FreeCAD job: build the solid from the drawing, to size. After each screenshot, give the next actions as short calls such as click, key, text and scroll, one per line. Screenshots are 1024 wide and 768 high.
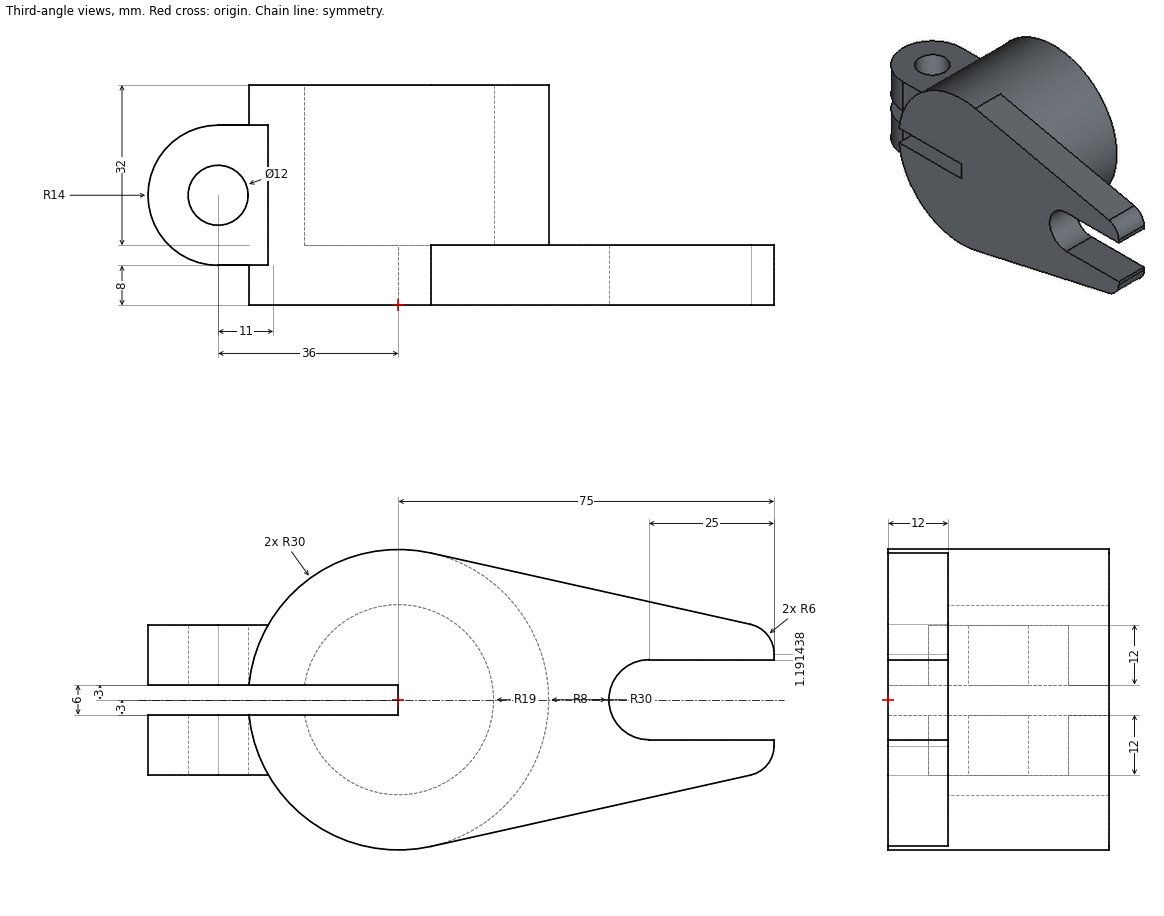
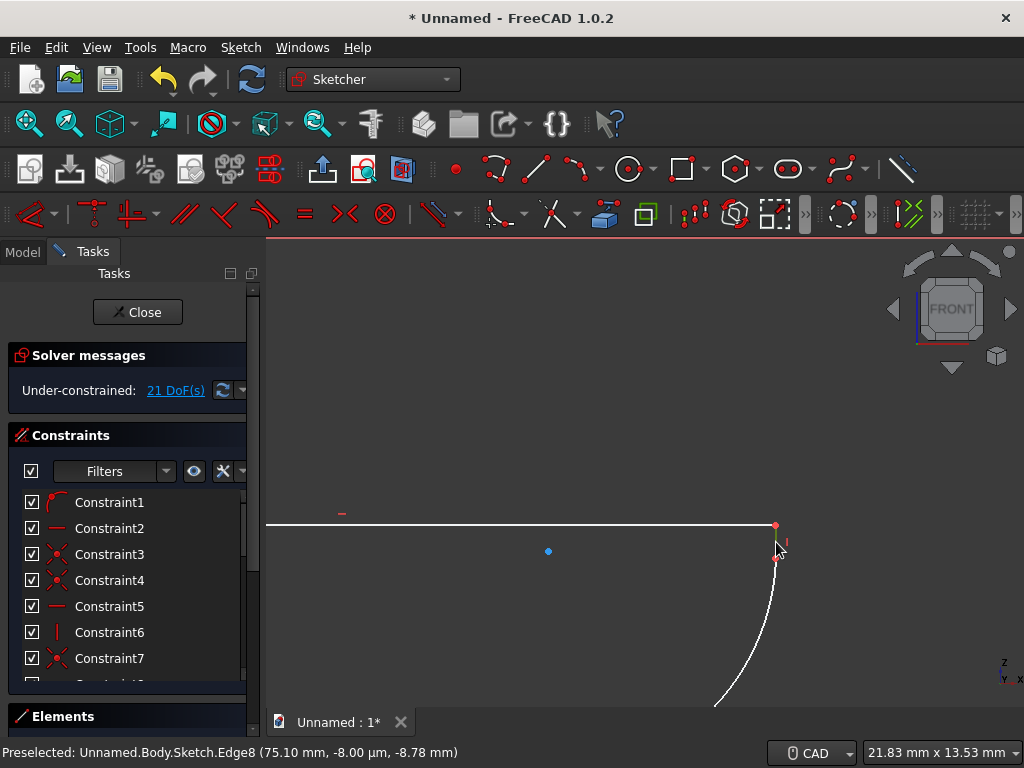
scroll(779, 501, down, 11)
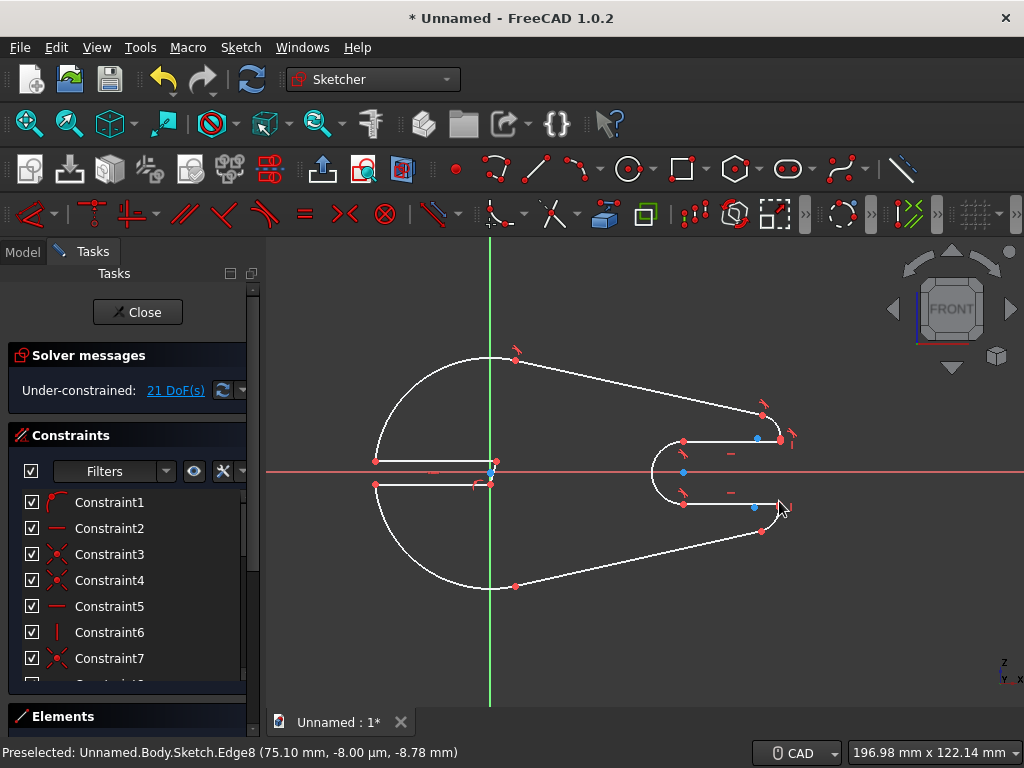
scroll(777, 517, up, 2)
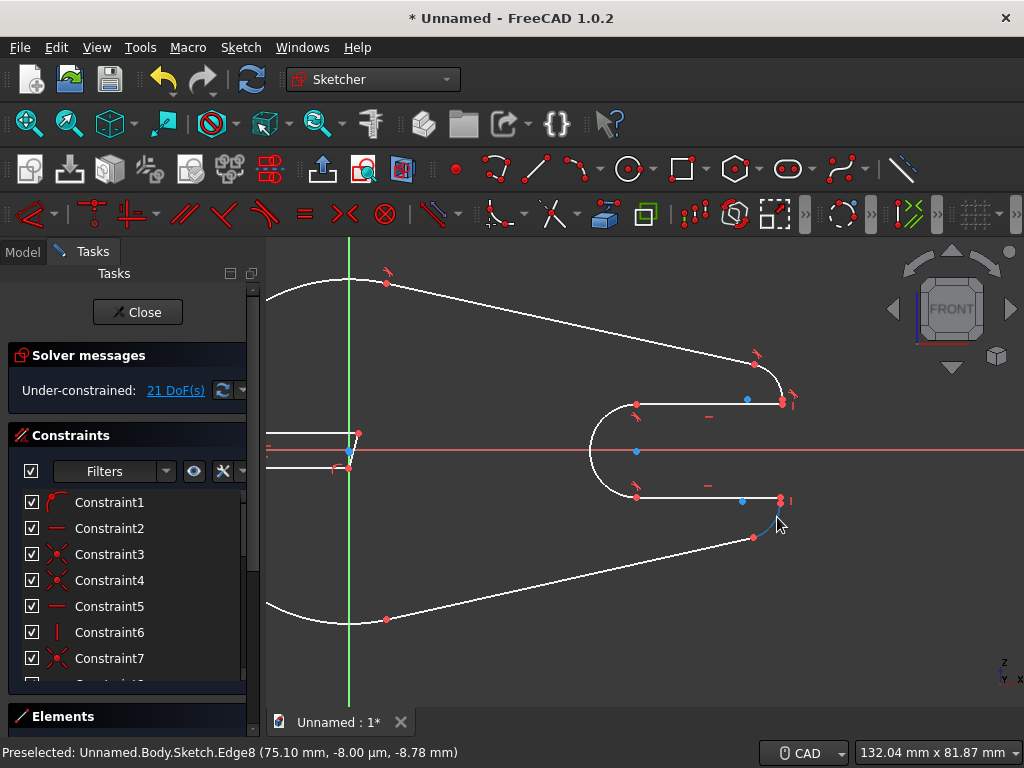
click(777, 517)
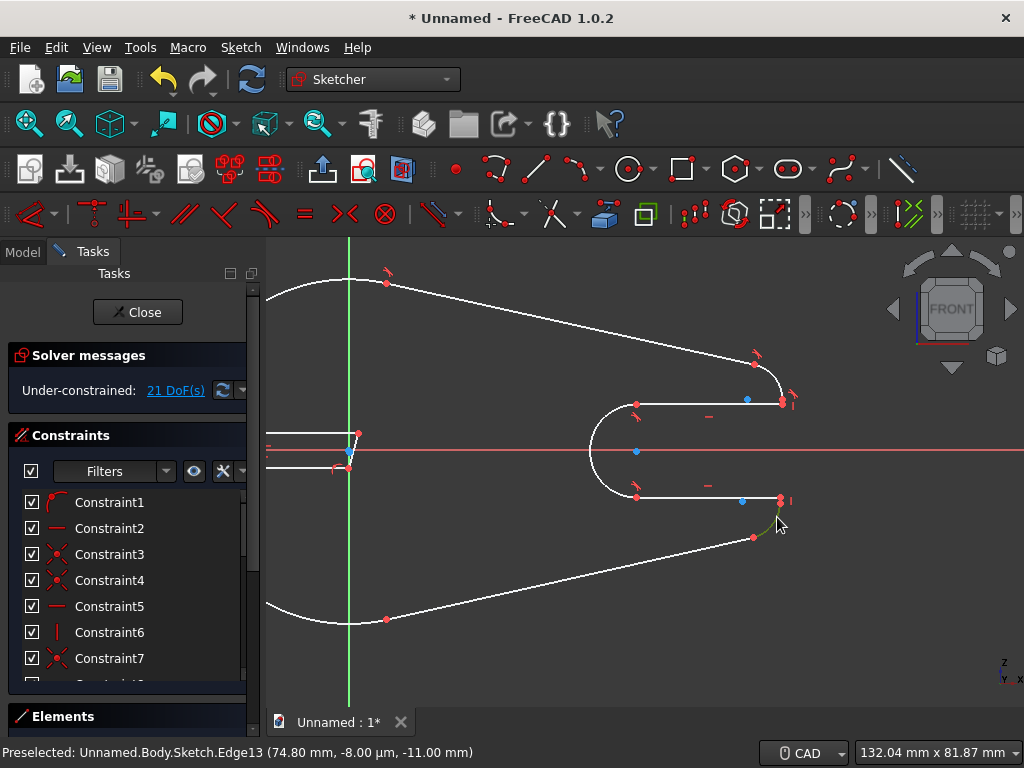
key(t)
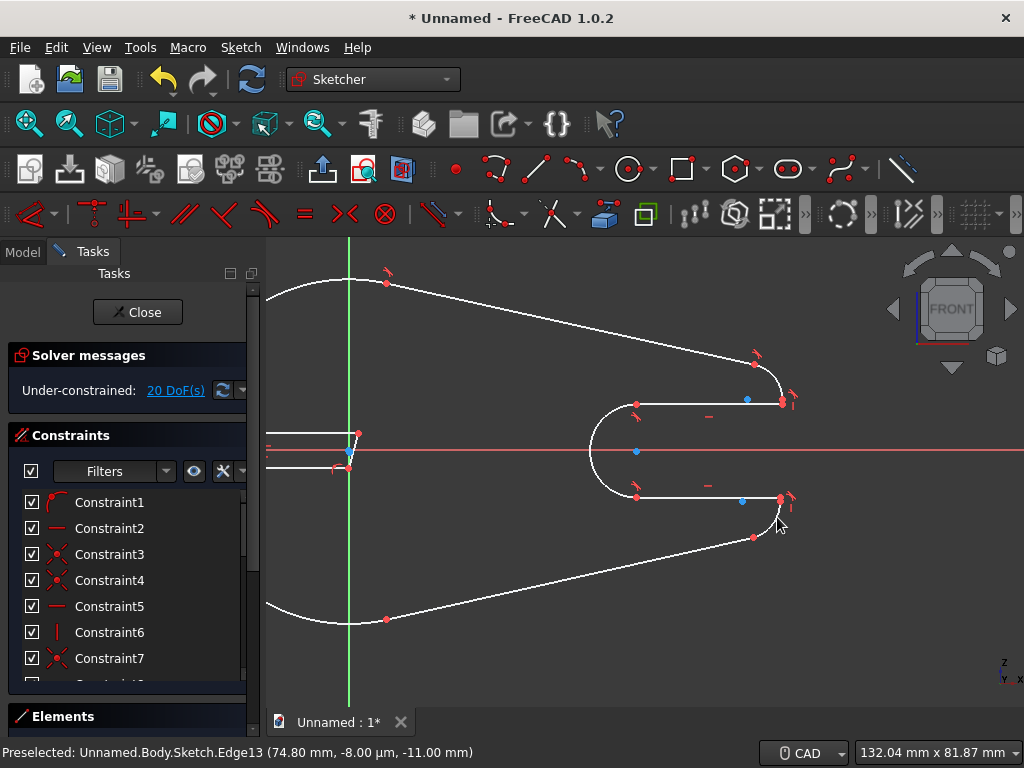
click(643, 562)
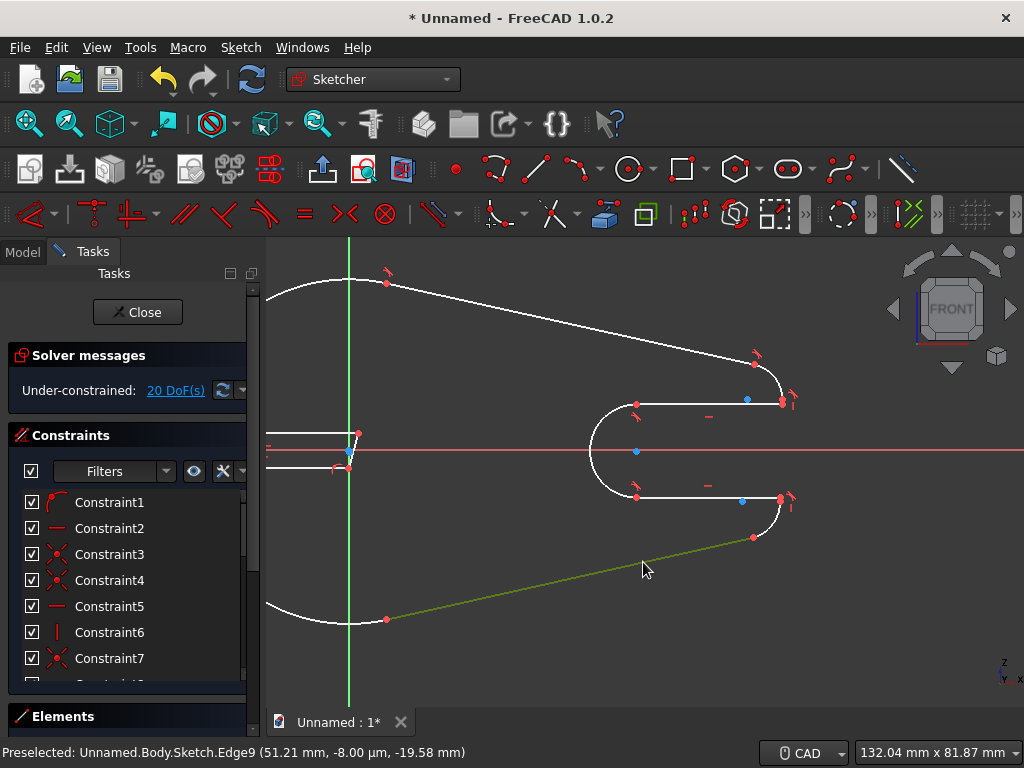
click(766, 531)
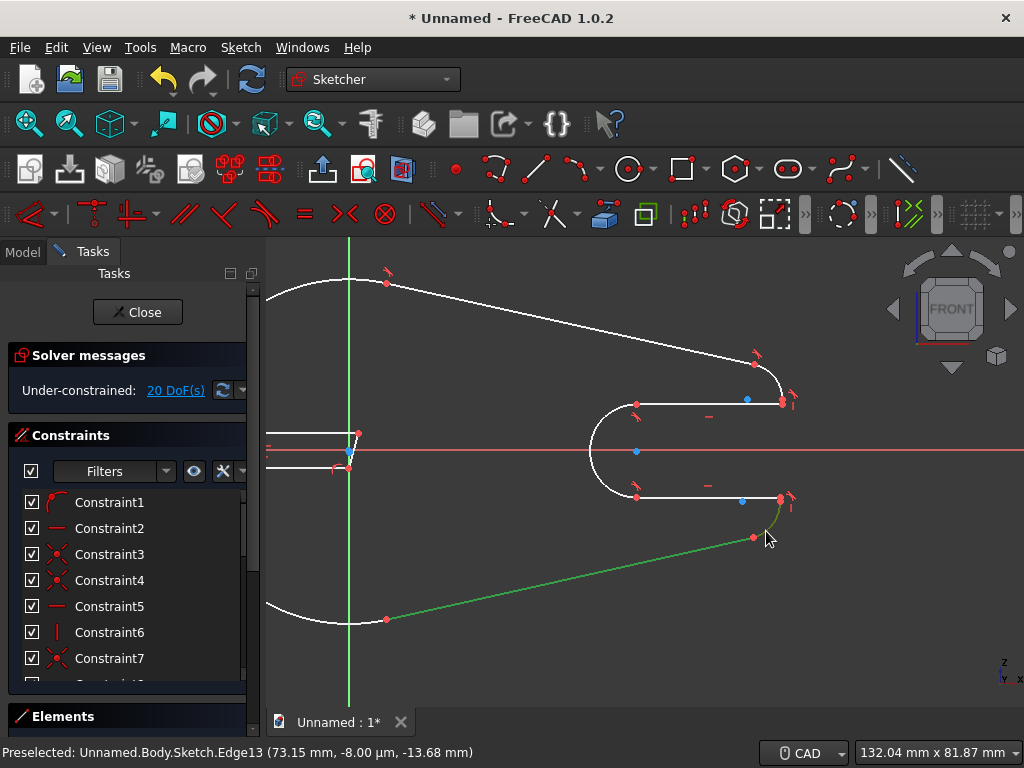
click(266, 214)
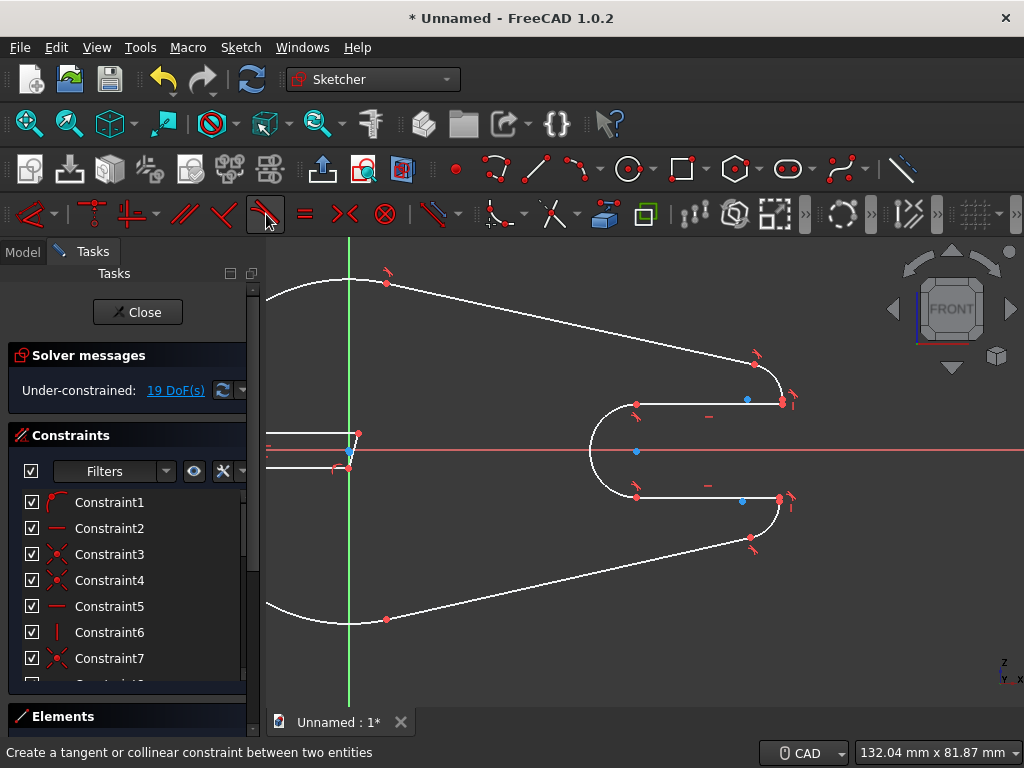
click(641, 562)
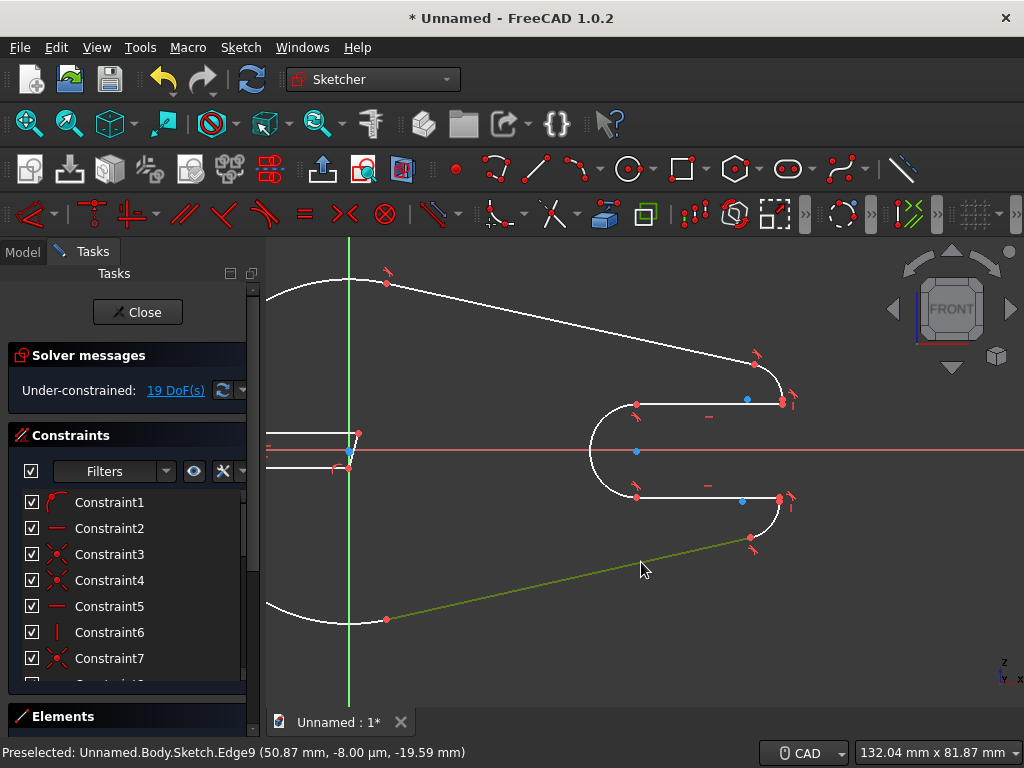
click(300, 617)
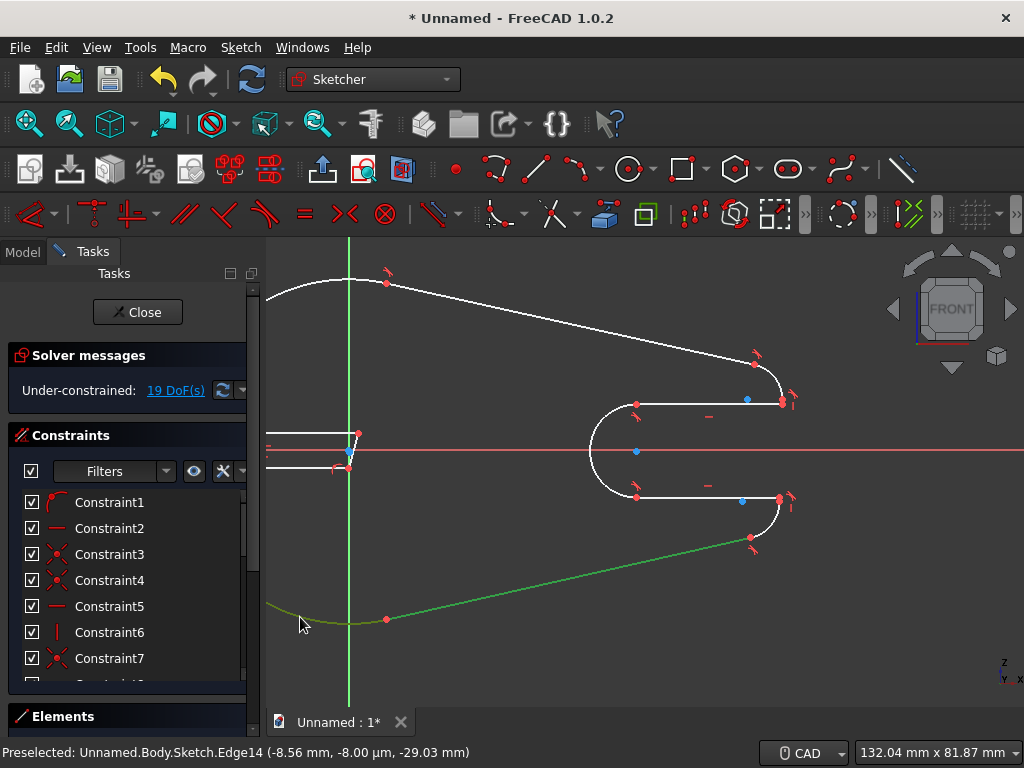
key(t)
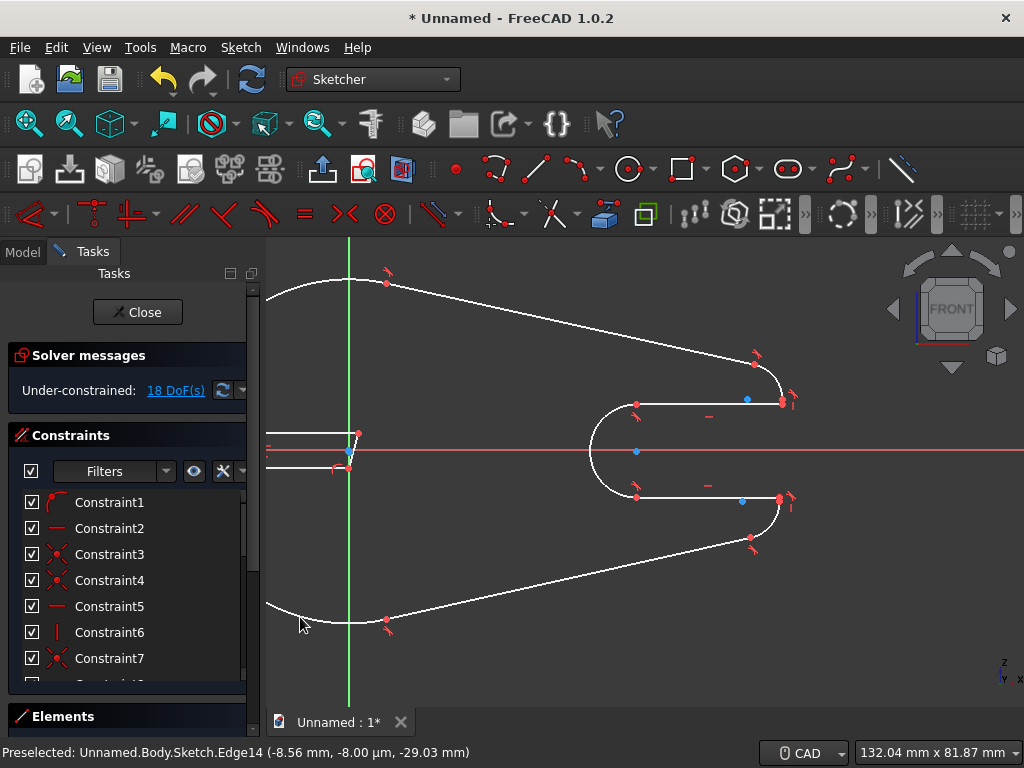
scroll(352, 458, up, 3)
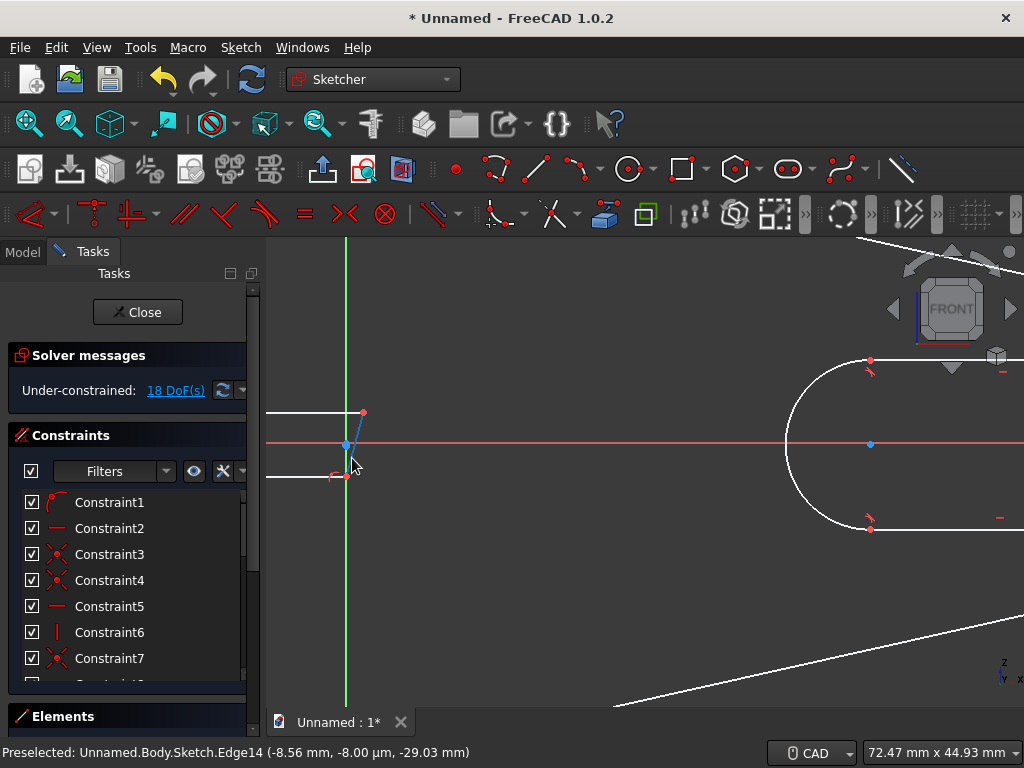
click(351, 458)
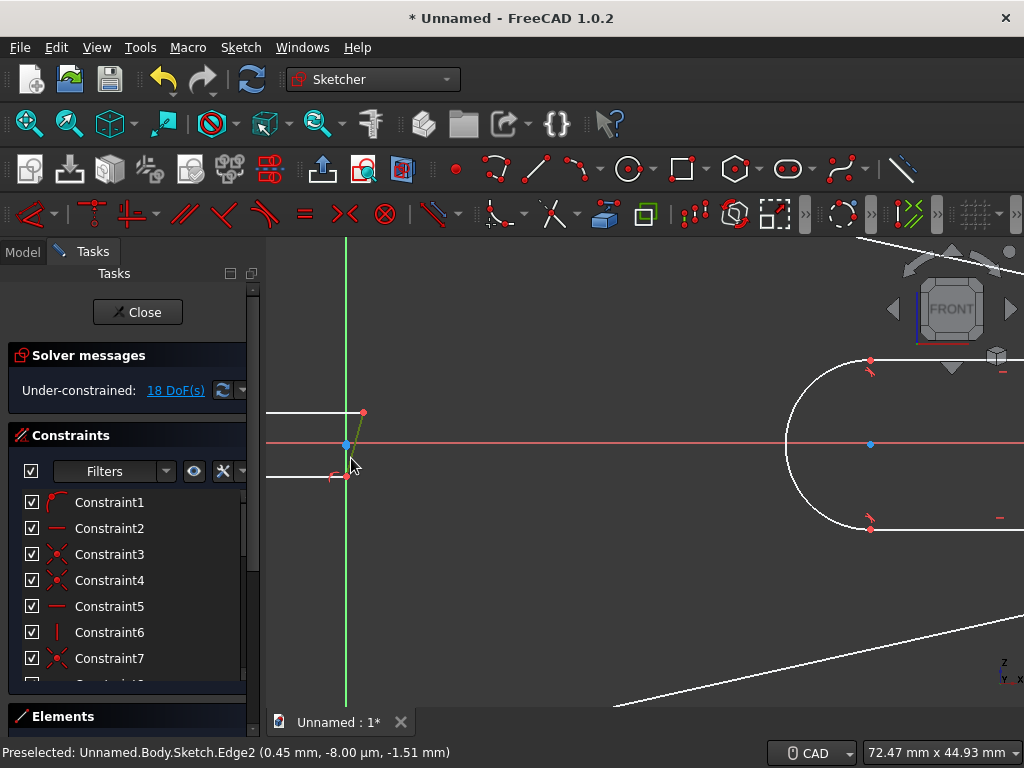
key(v)